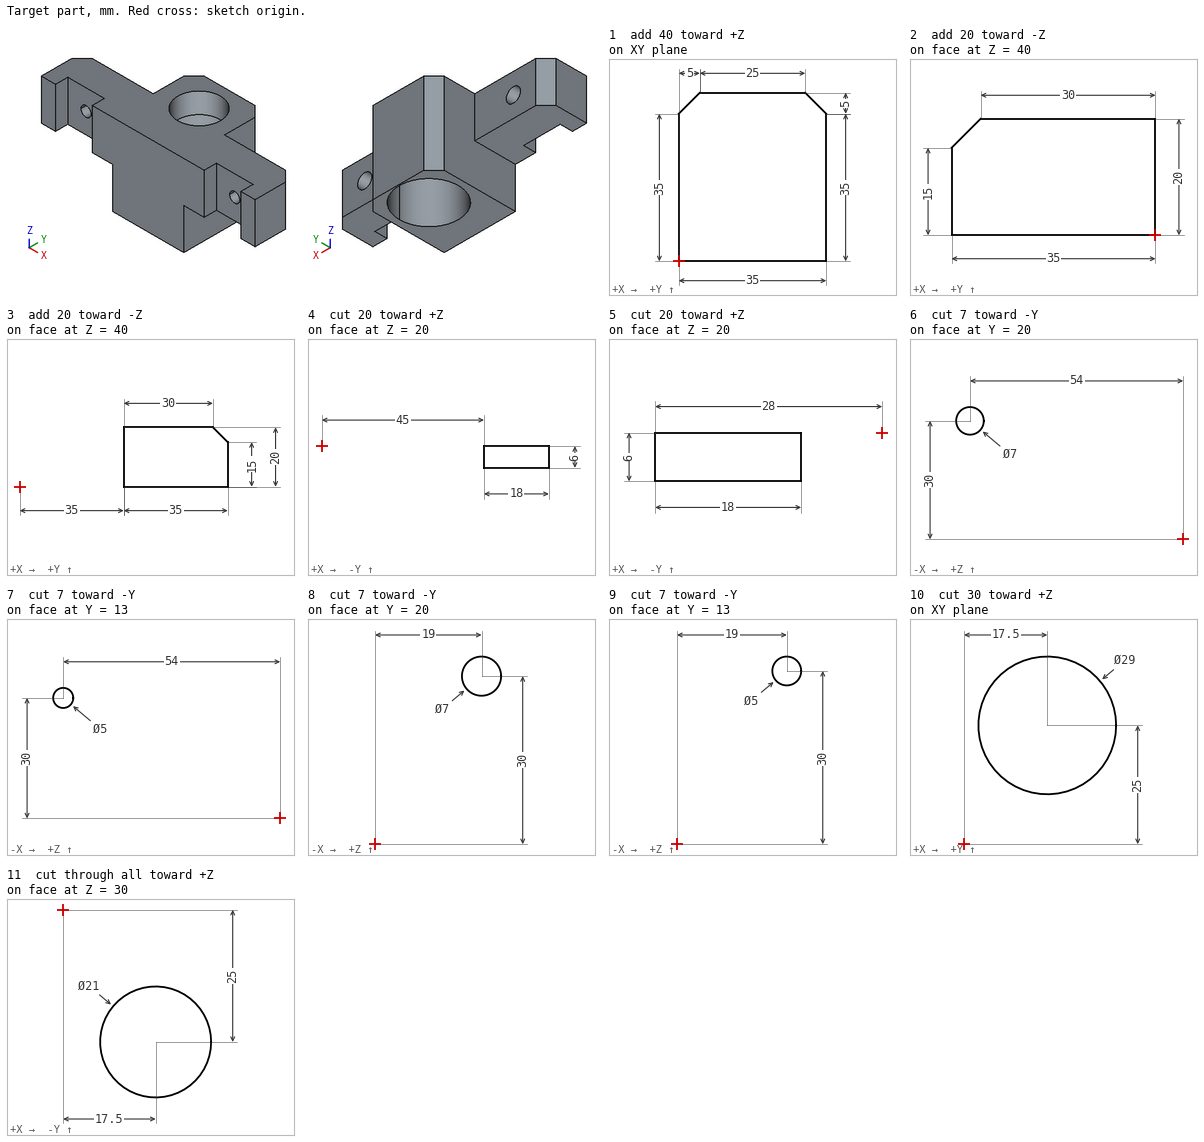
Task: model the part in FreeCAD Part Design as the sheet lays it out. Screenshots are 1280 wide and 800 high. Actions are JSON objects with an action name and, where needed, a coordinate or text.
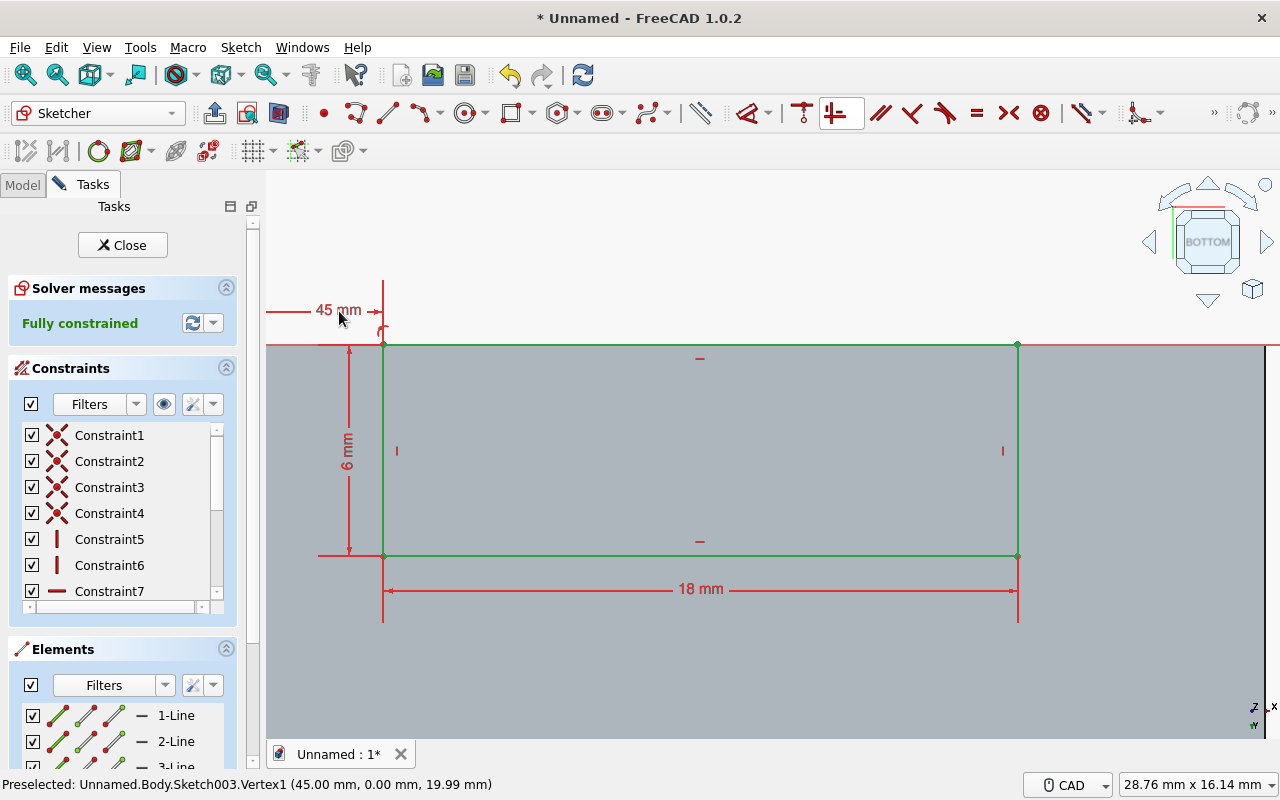
{"action": "left_click", "coordinate": [123, 245]}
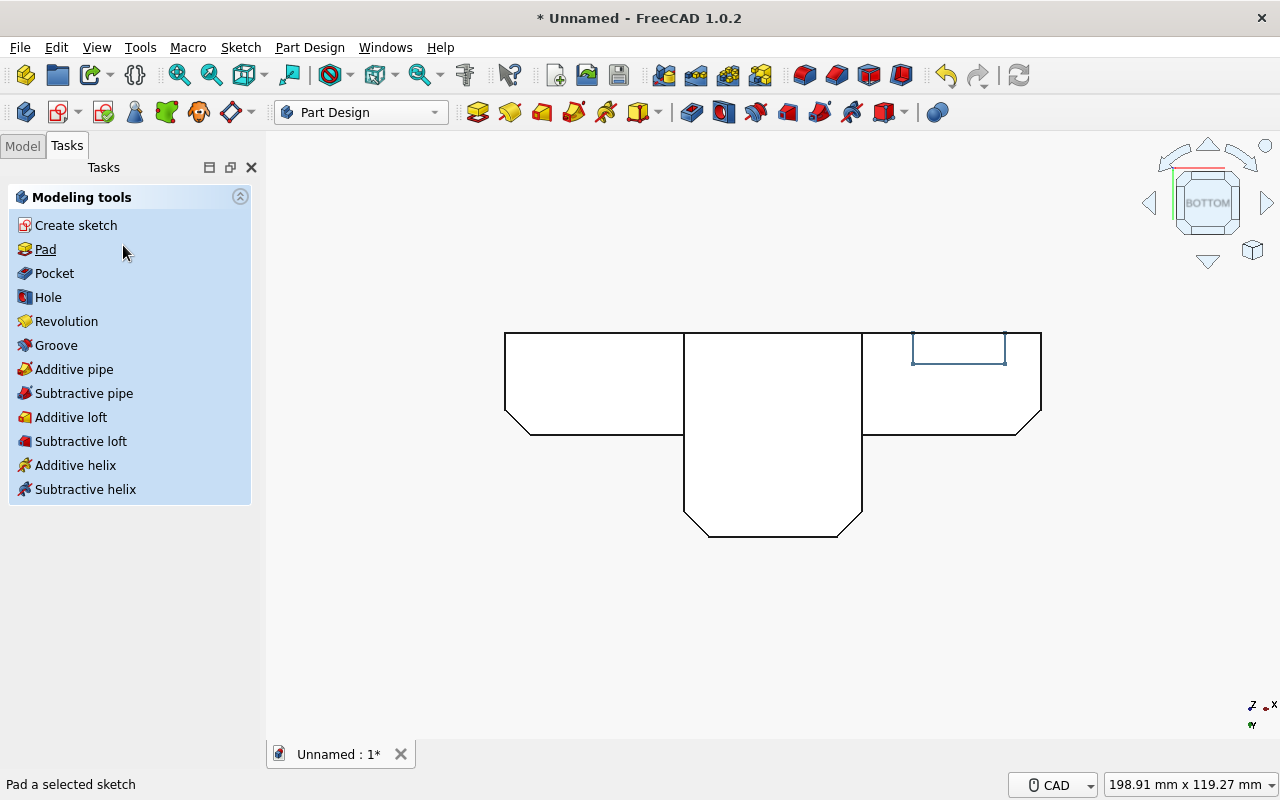
{"action": "left_click", "coordinate": [692, 112]}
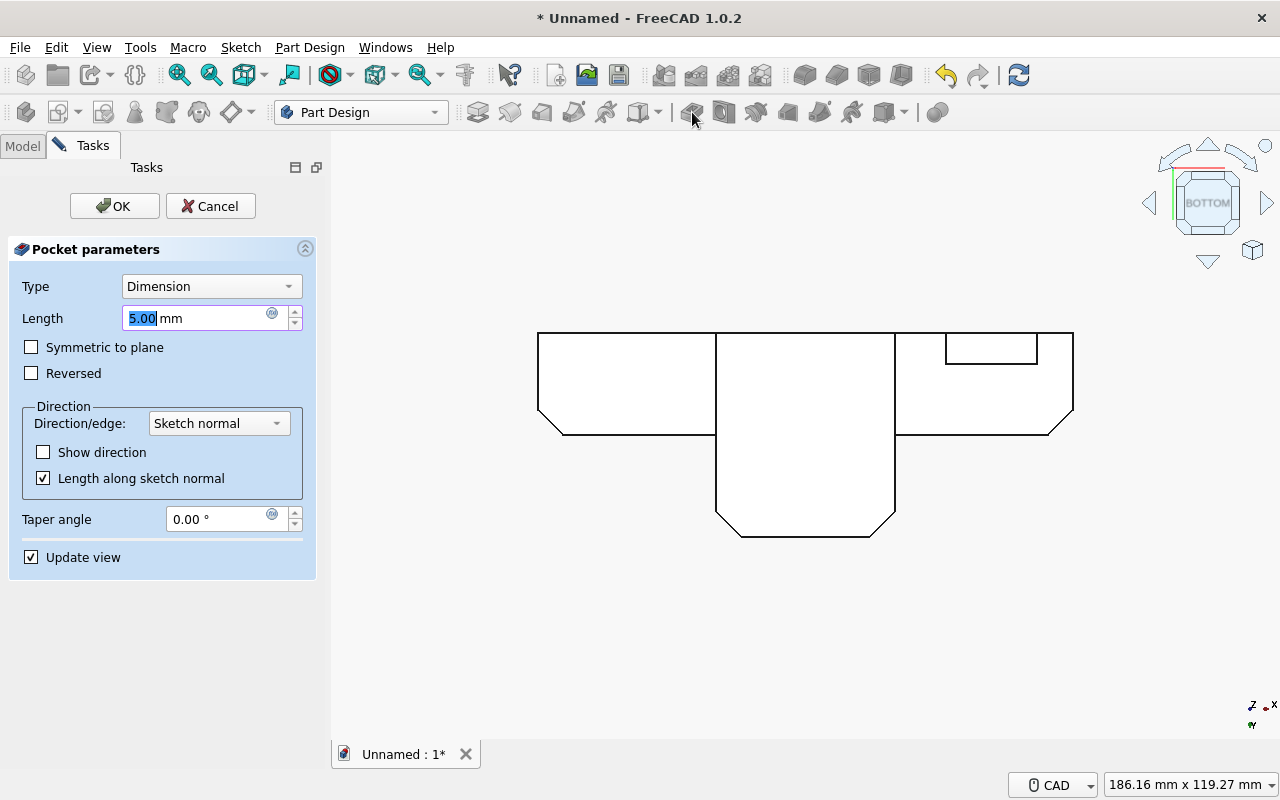
{"action": "type", "text": "20"}
{"action": "key", "text": "Tab"}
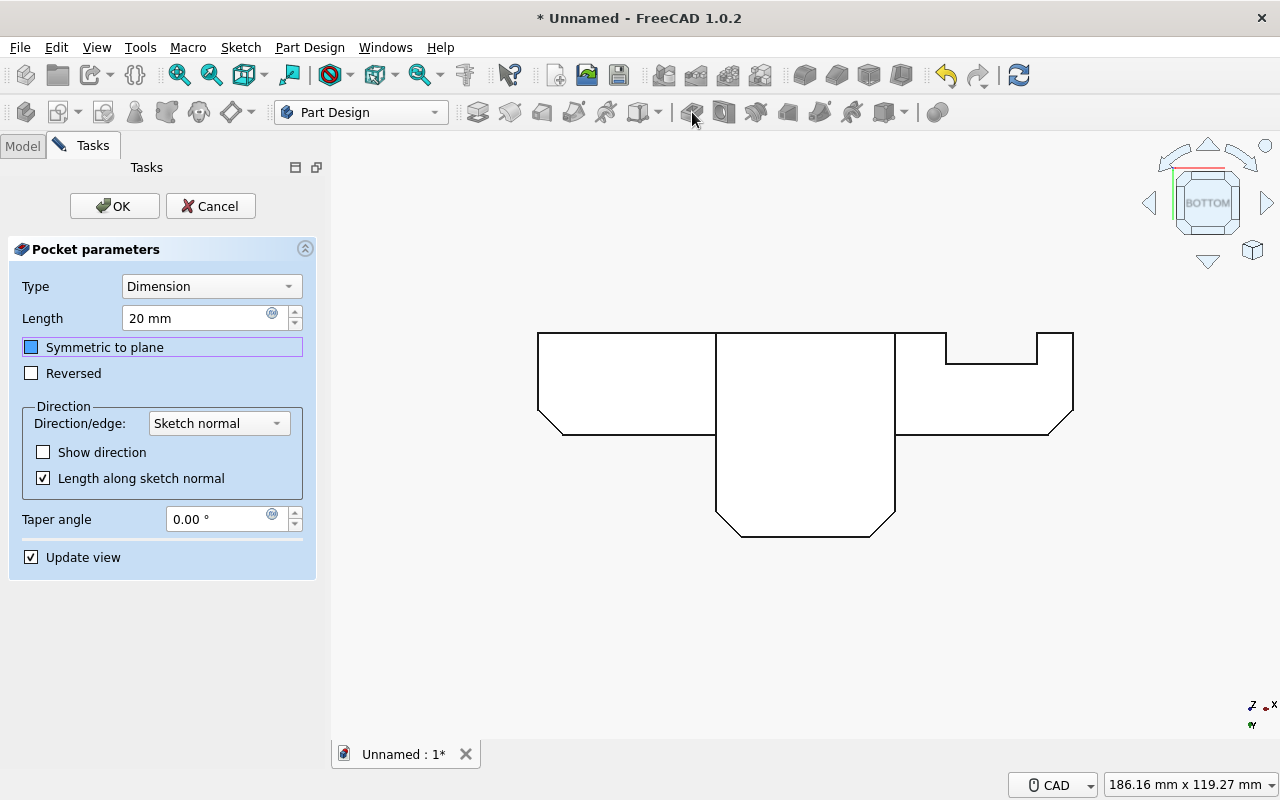
{"action": "left_click", "coordinate": [115, 206]}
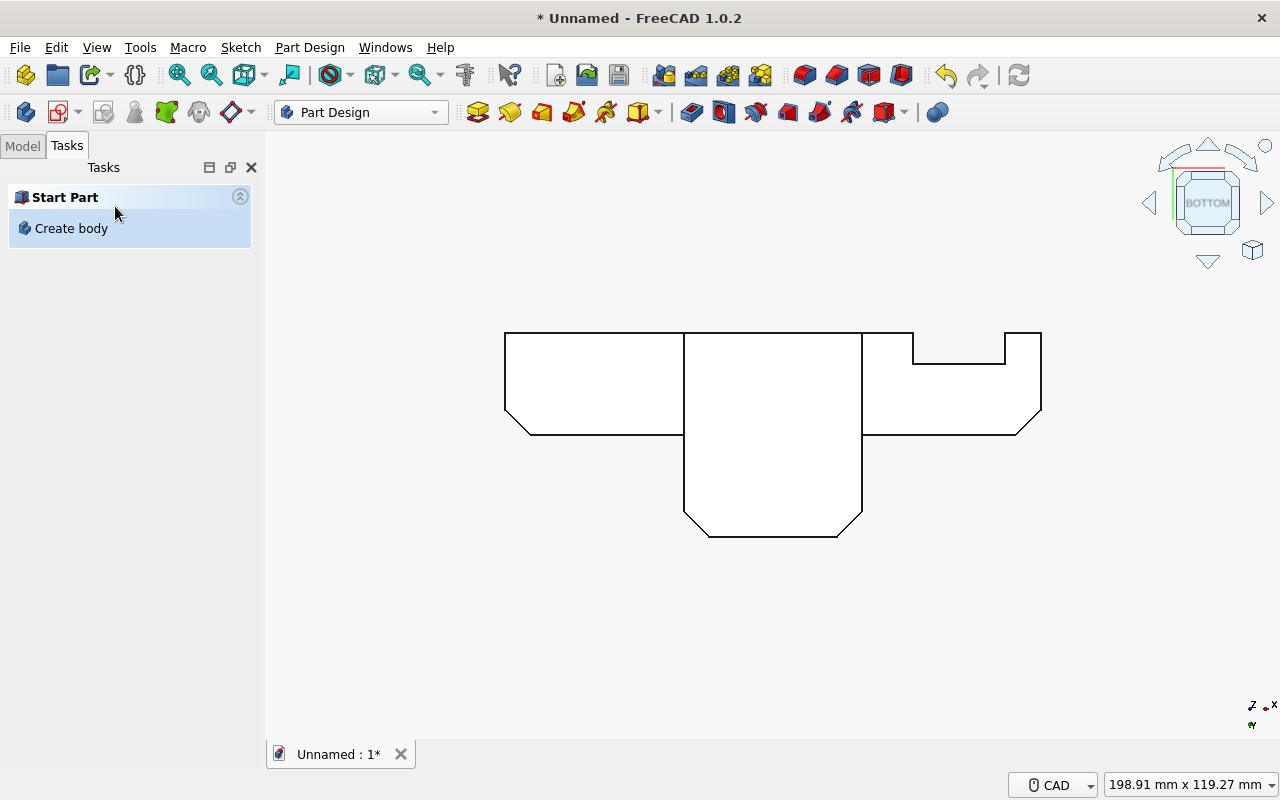
{"action": "left_click", "coordinate": [620, 383]}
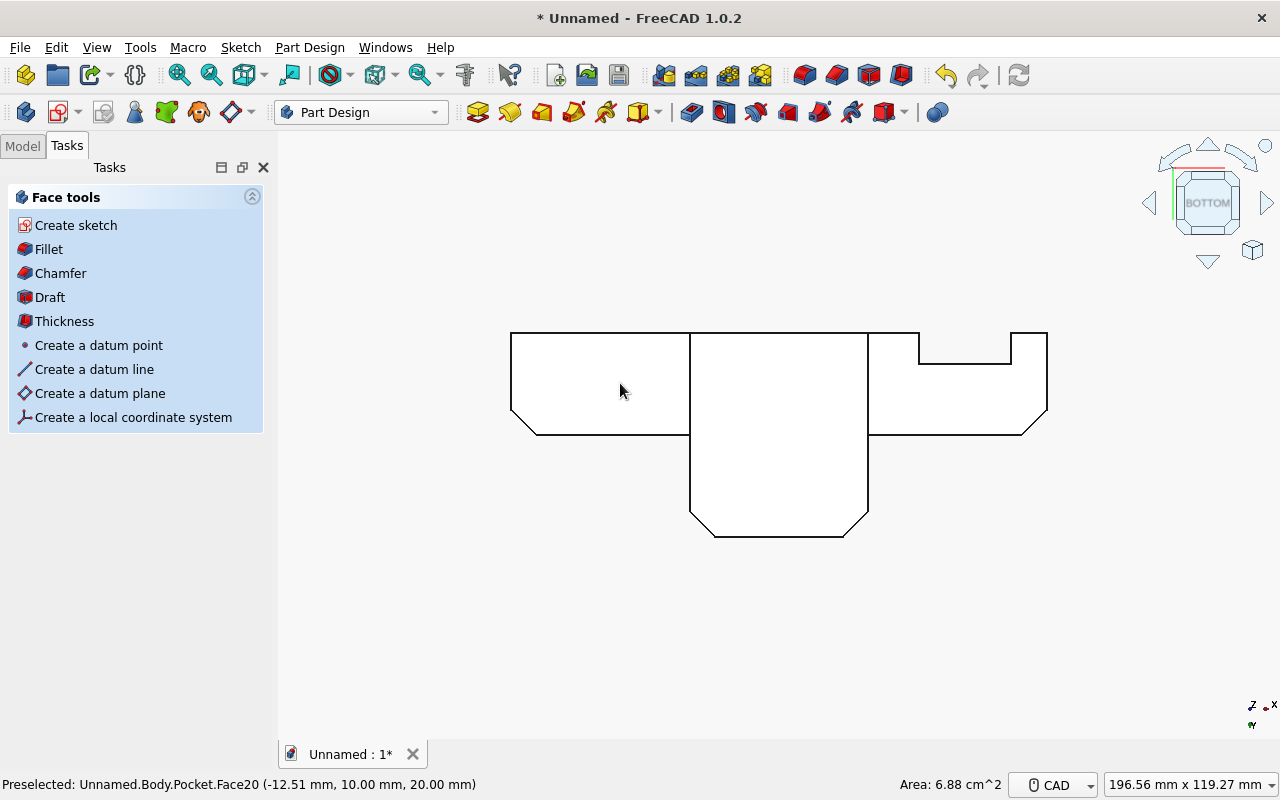
{"action": "left_click", "coordinate": [58, 112]}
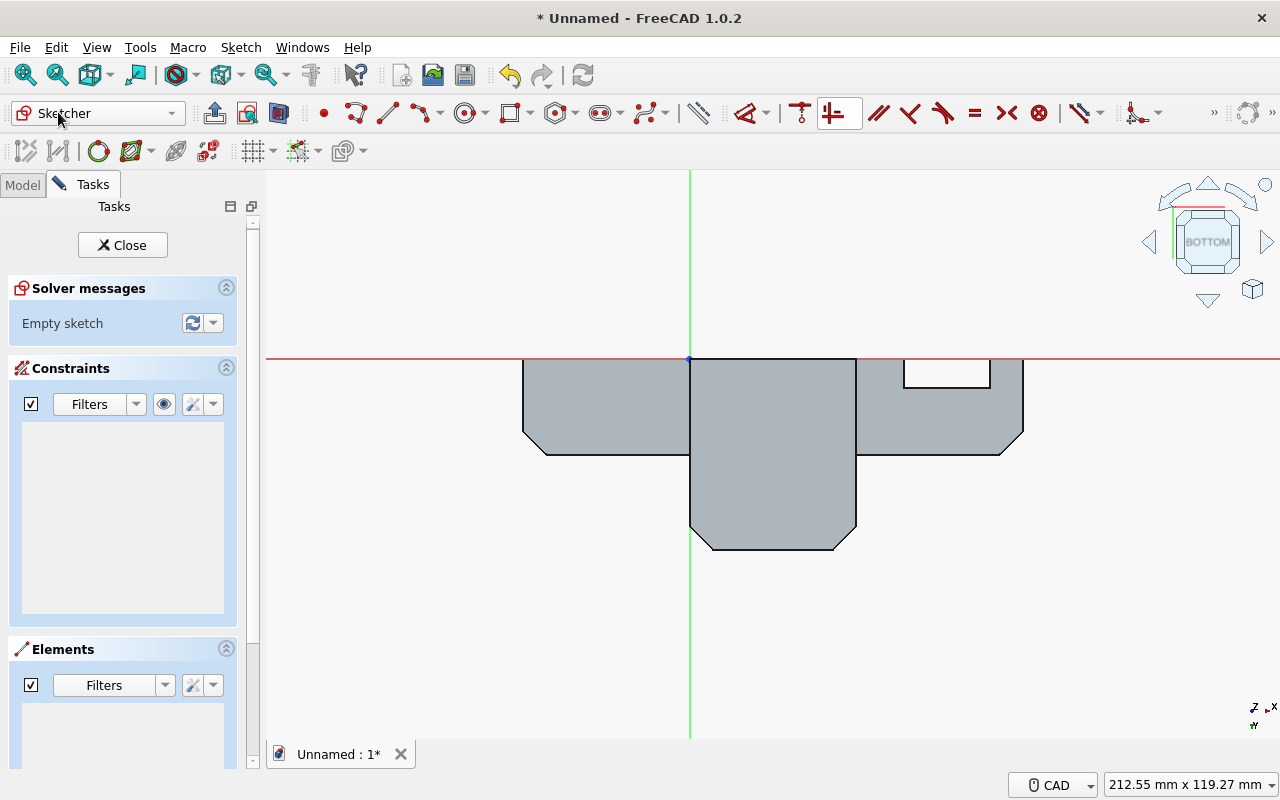
{"action": "scroll", "coordinate": [596, 347], "scroll_direction": "up", "scroll_amount": 7}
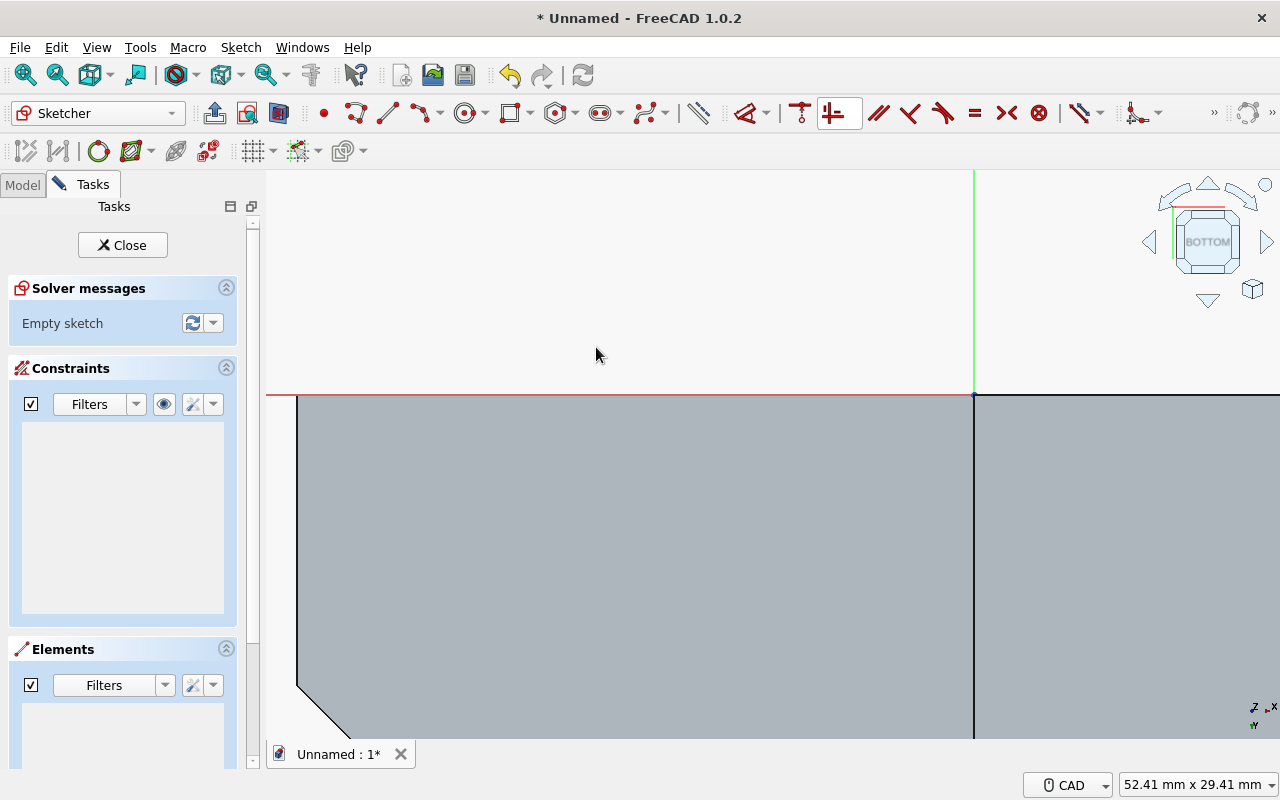
{"action": "left_click", "coordinate": [510, 114]}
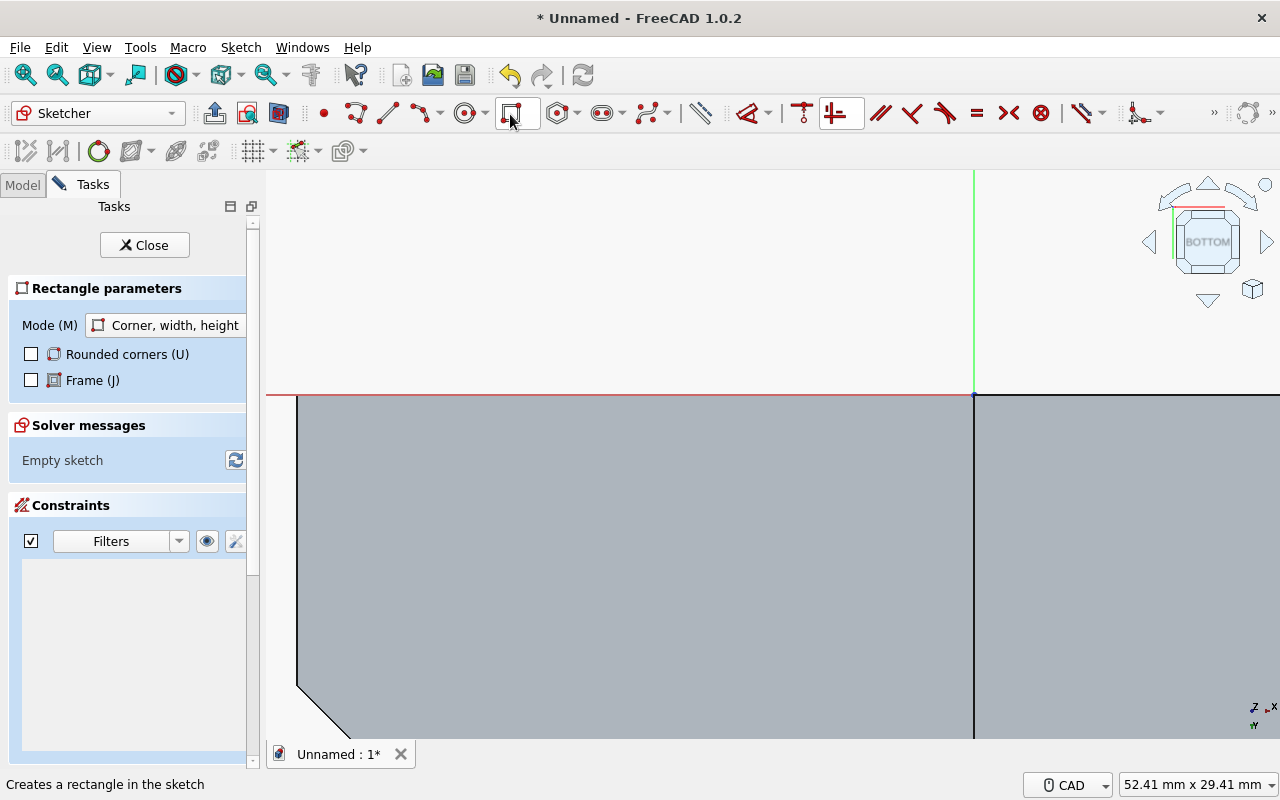
{"action": "left_click", "coordinate": [433, 395]}
{"action": "left_click", "coordinate": [781, 511]}
{"action": "key", "text": "Escape"}